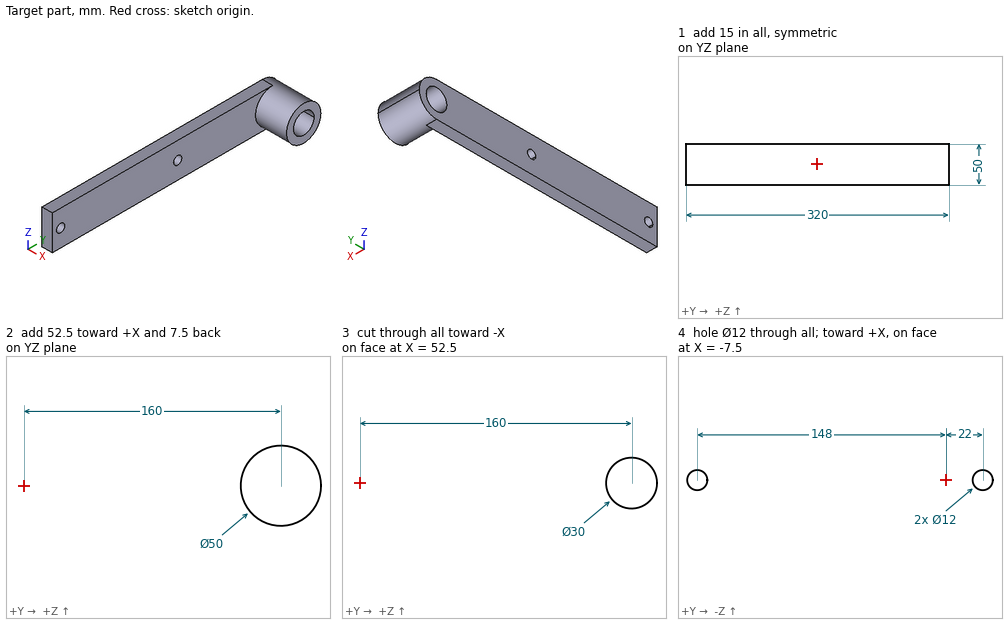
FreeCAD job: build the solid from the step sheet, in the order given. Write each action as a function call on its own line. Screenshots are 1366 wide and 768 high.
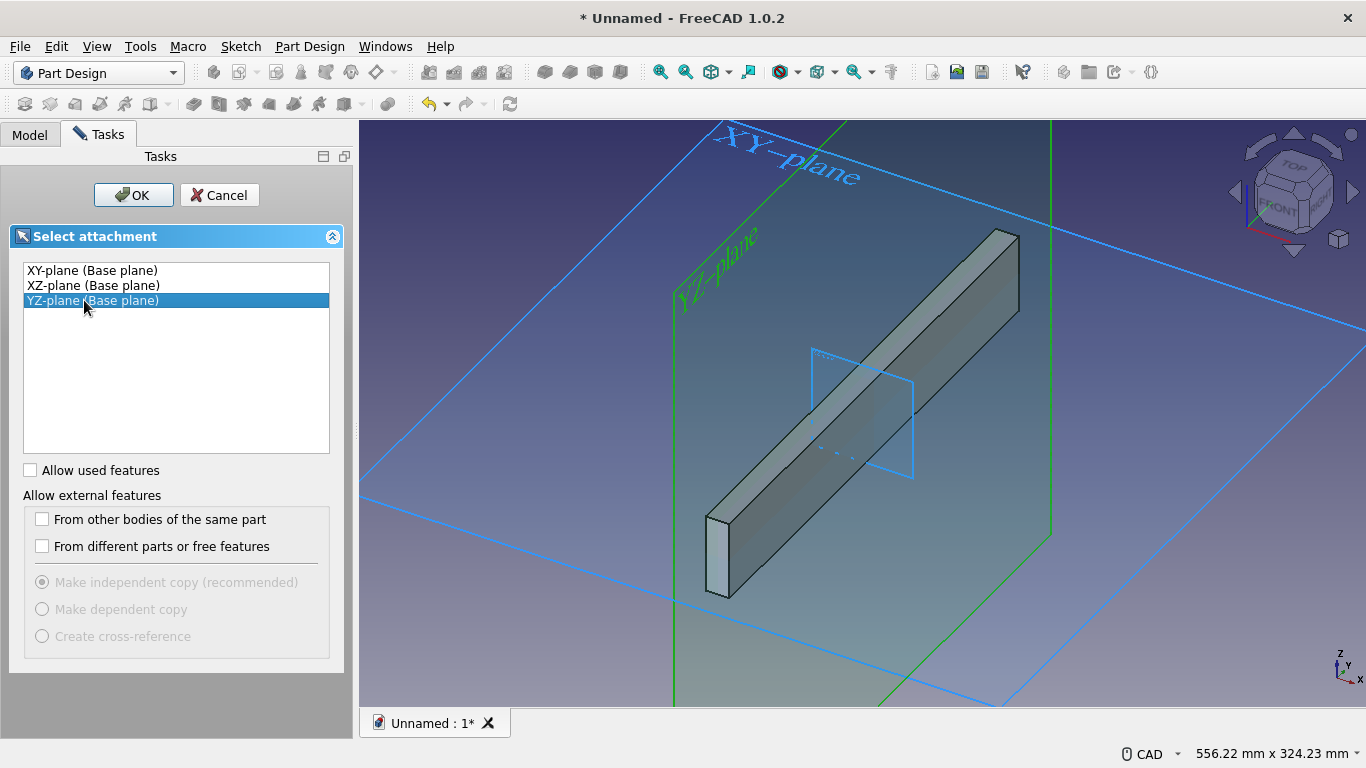
click(134, 195)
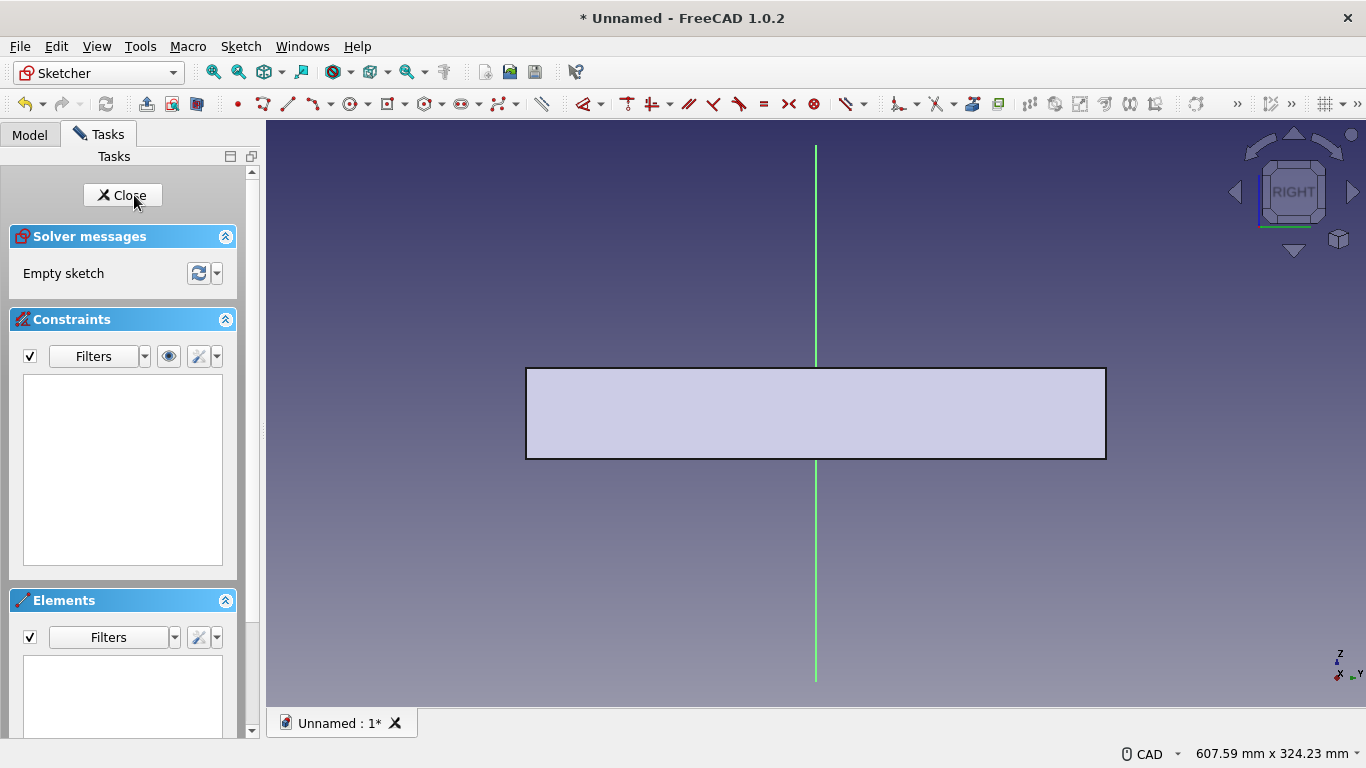
click(197, 104)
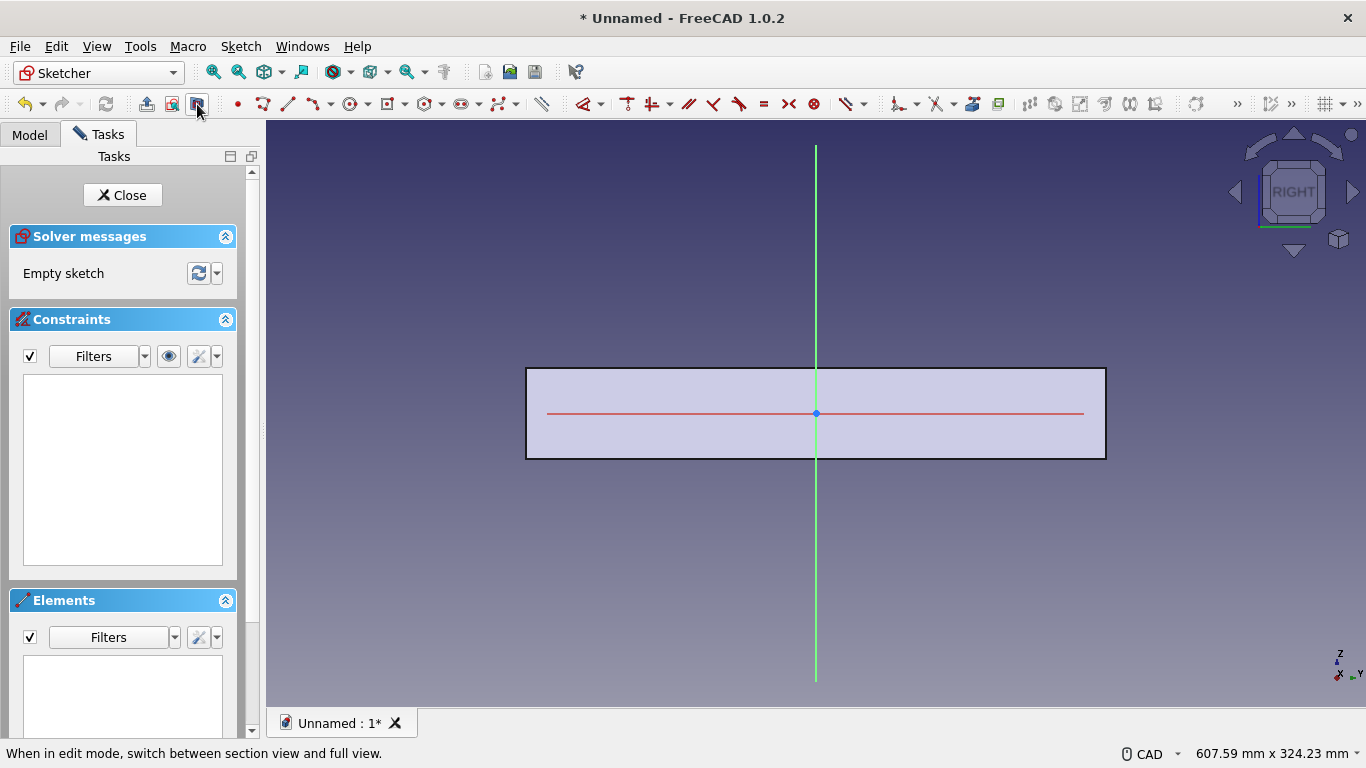
scroll(1201, 414, up, 7)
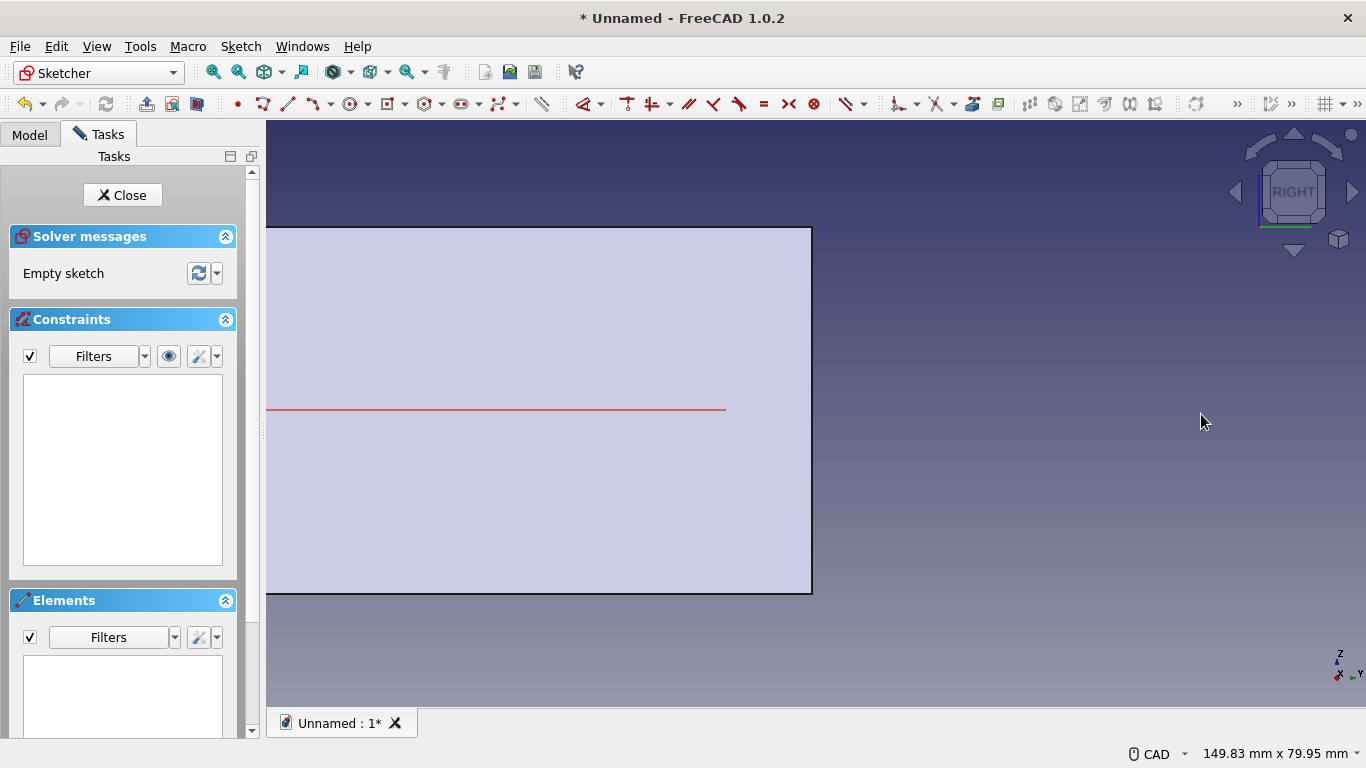
click(350, 104)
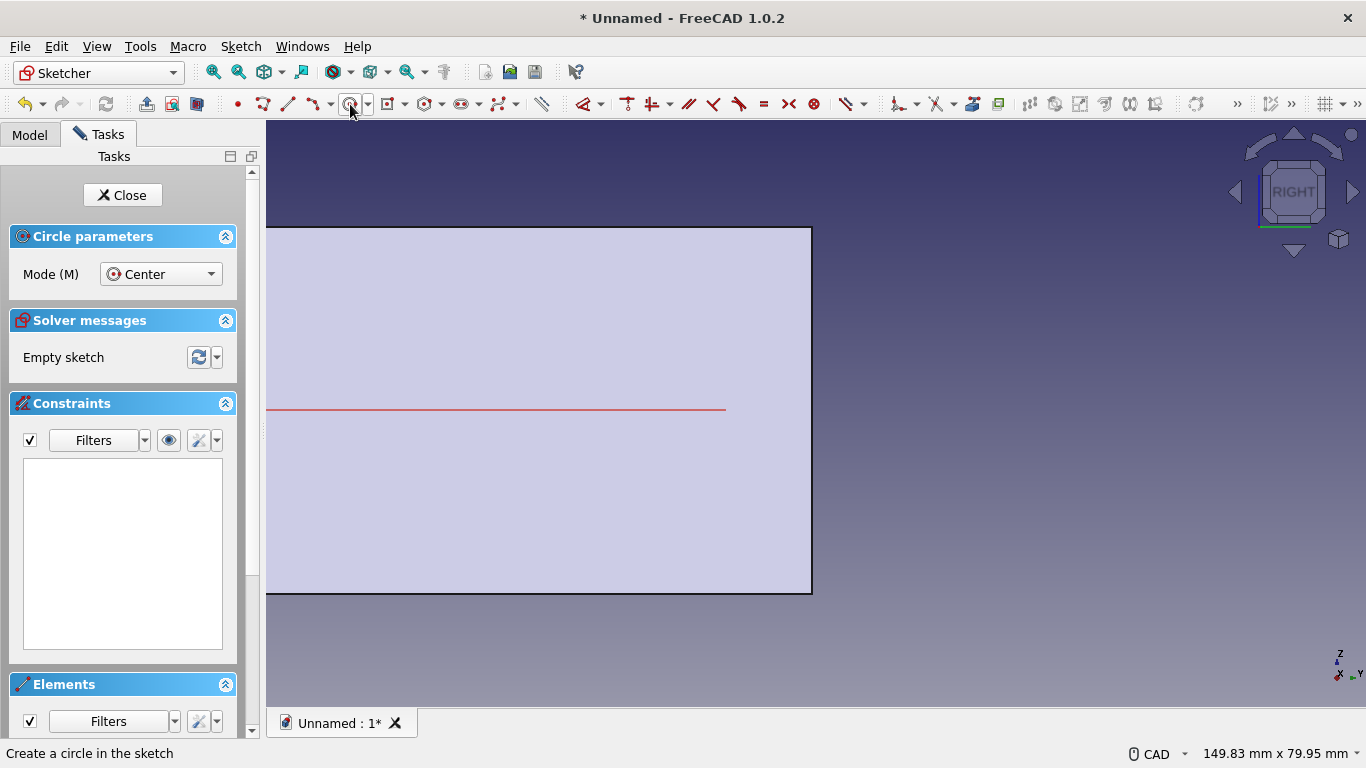
click(812, 410)
click(942, 281)
key(Escape)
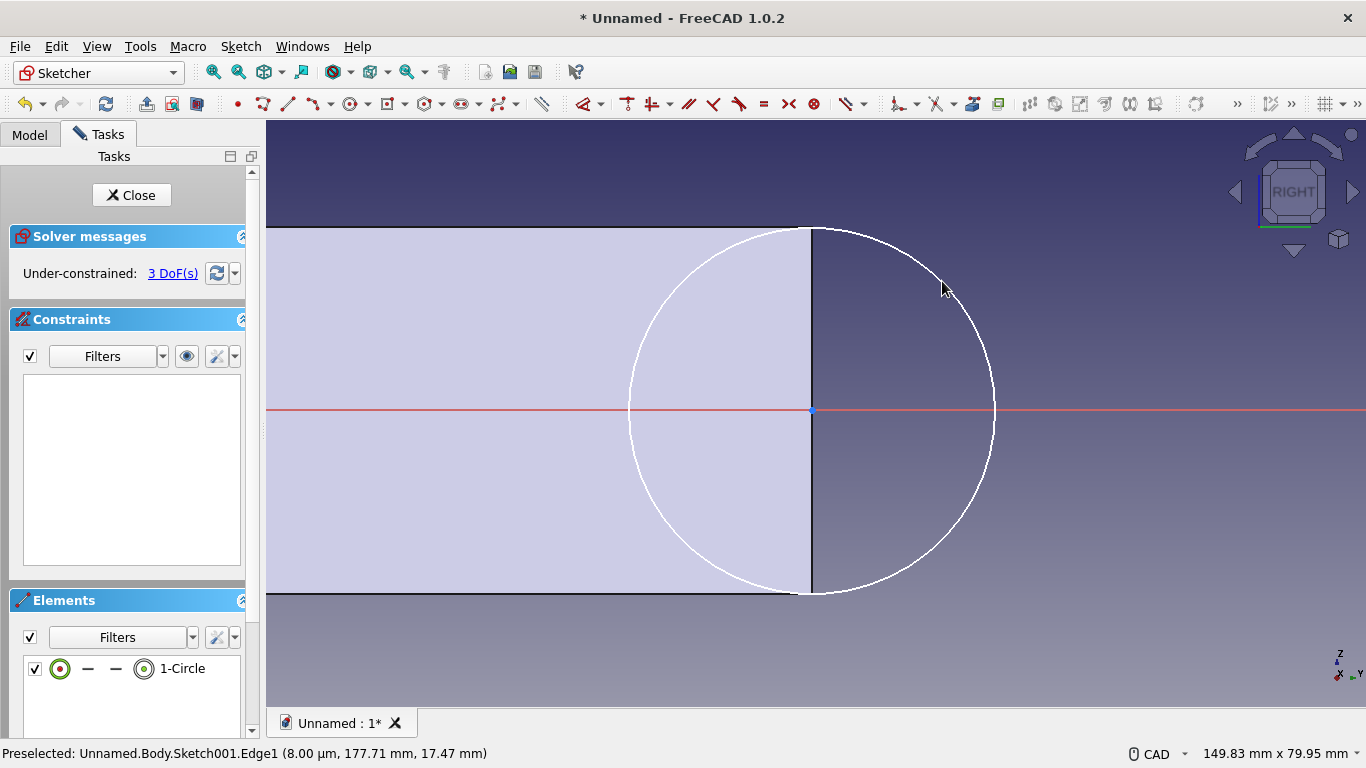
click(812, 411)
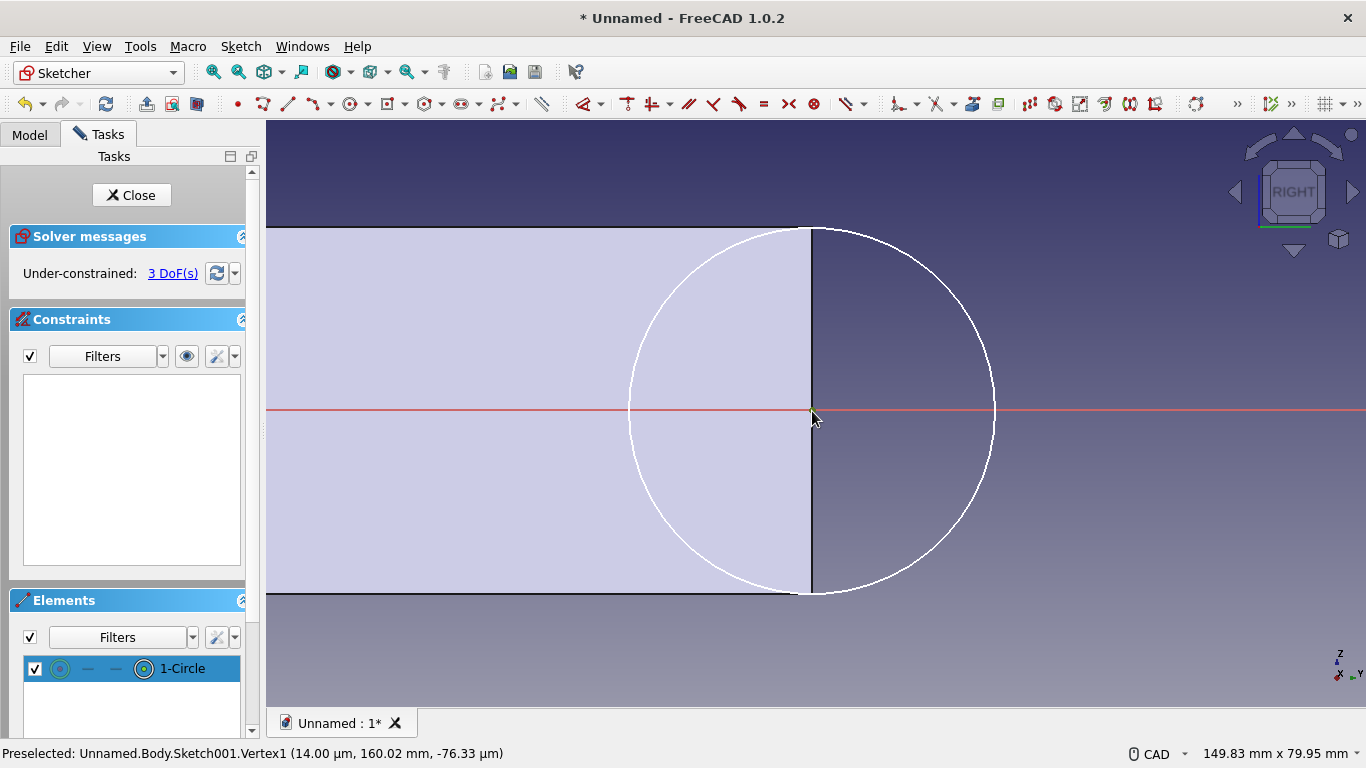
click(359, 410)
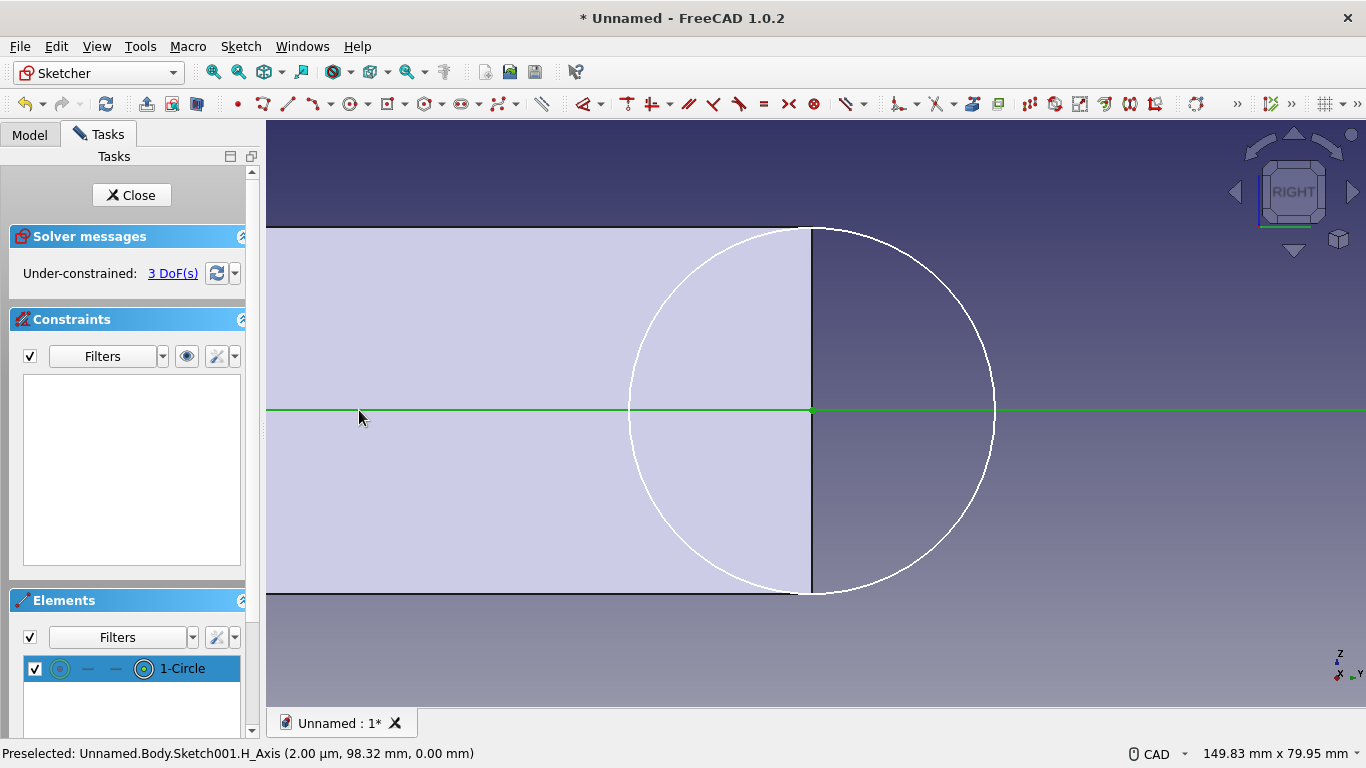
click(627, 104)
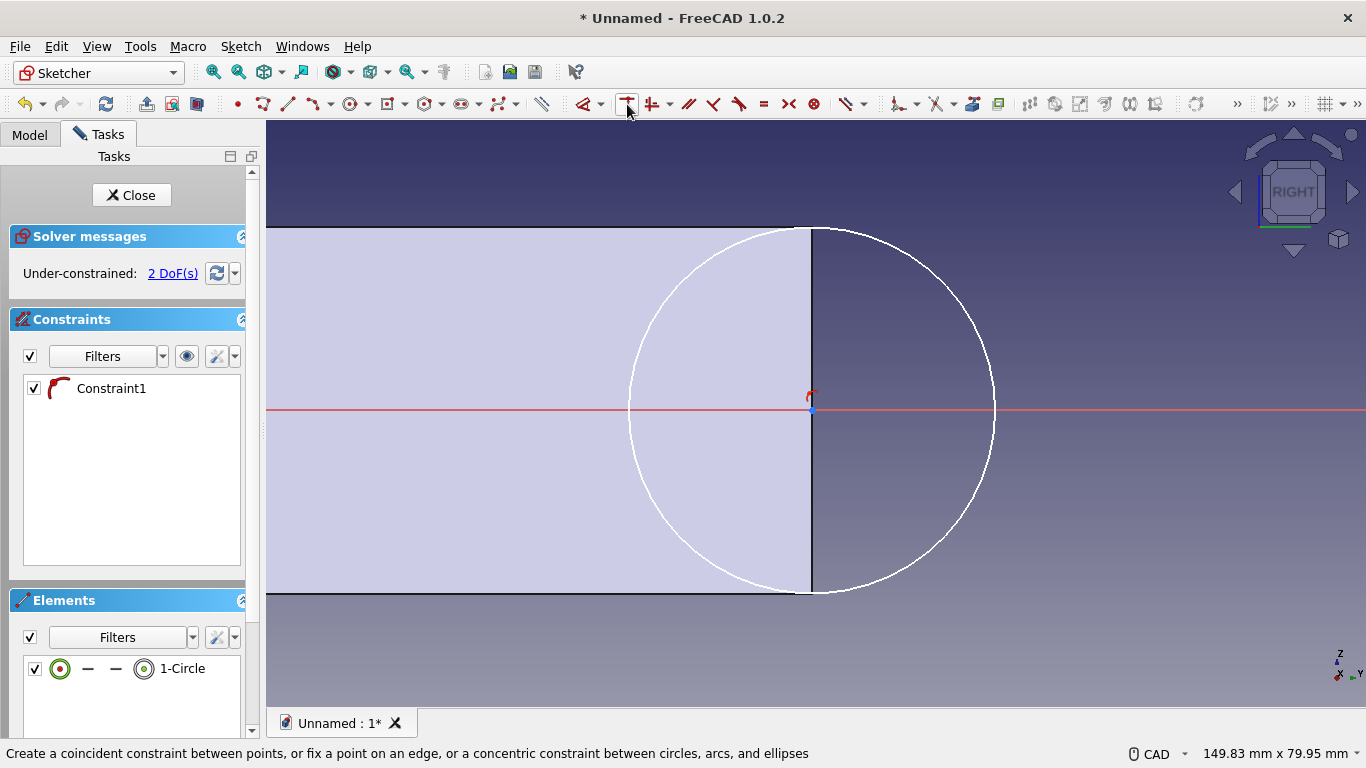
click(582, 104)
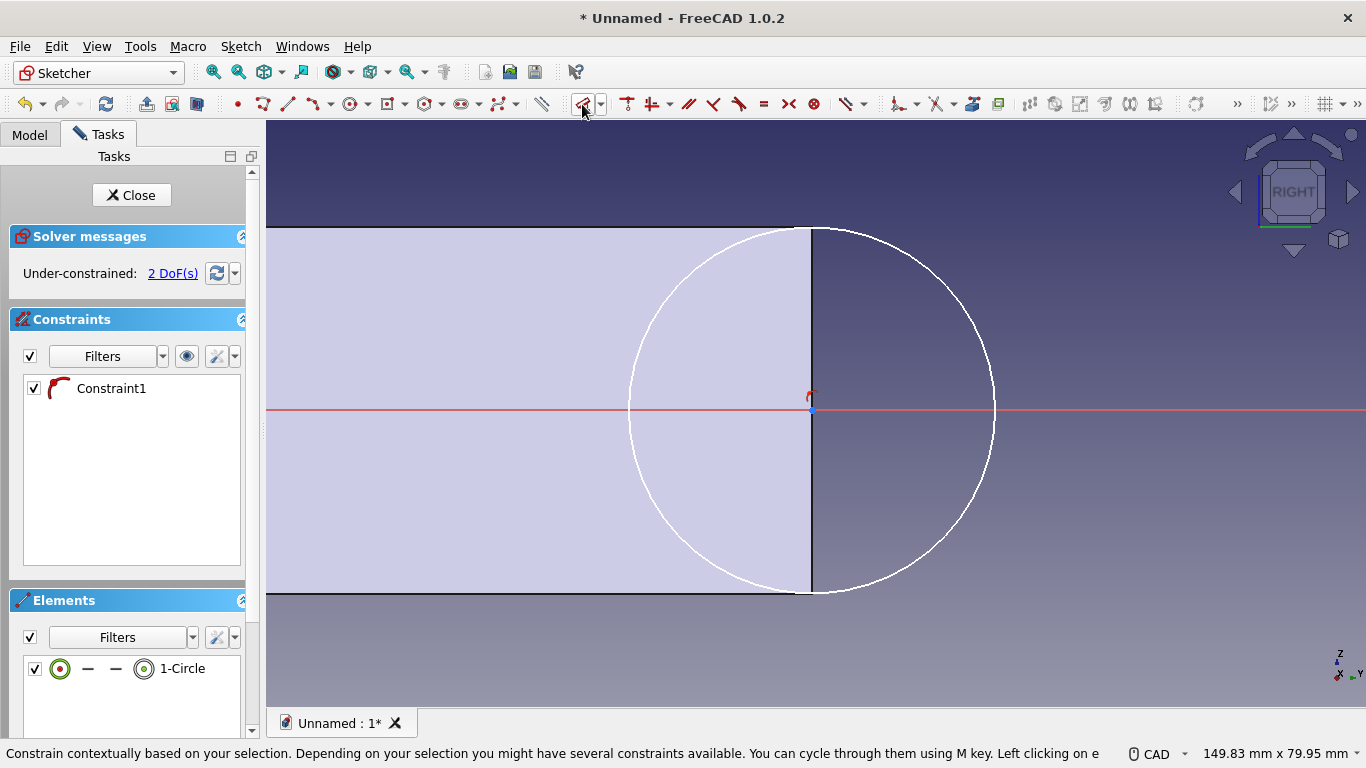
click(941, 281)
click(964, 258)